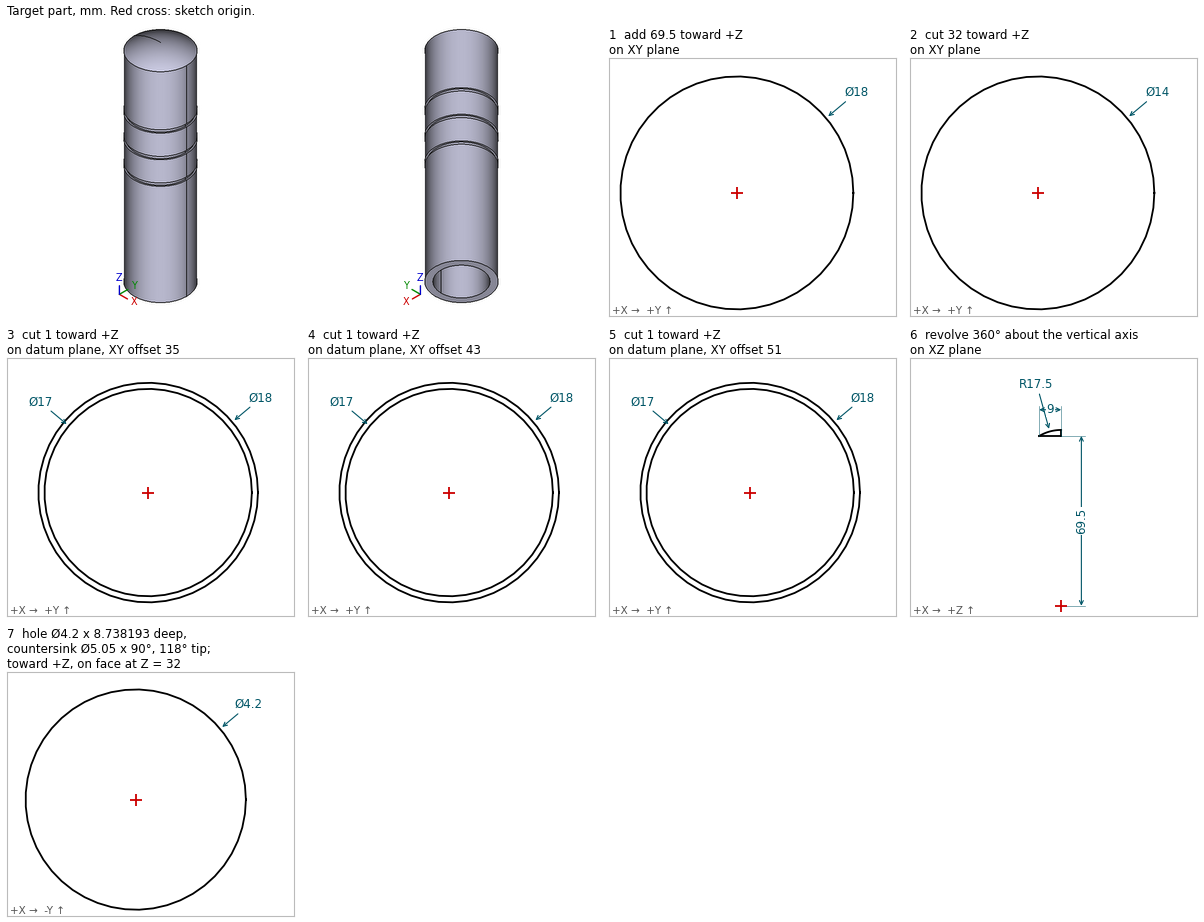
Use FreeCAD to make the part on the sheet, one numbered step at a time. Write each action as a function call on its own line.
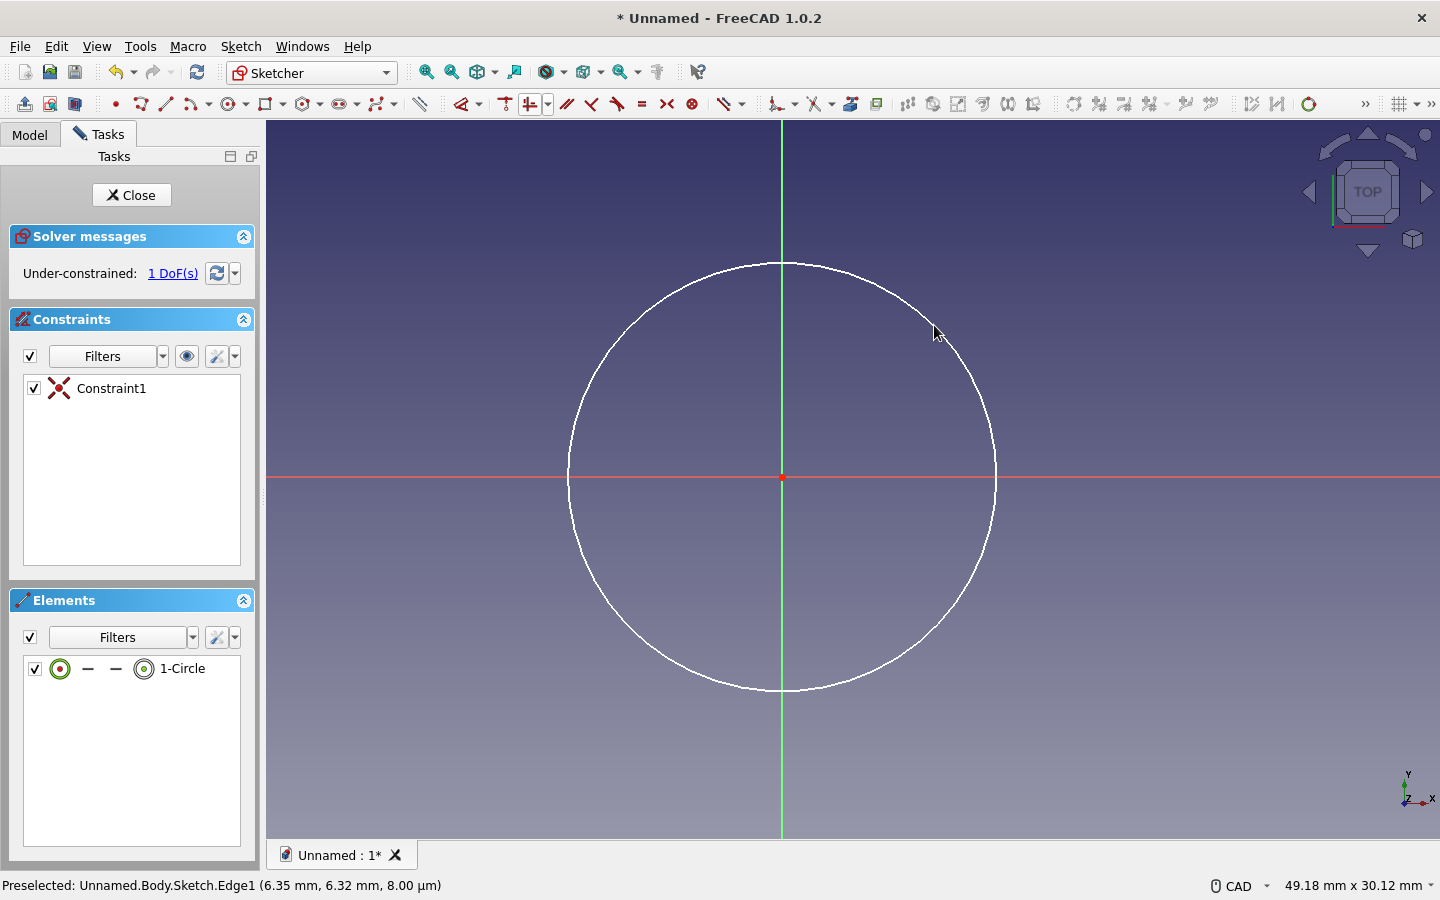
click(460, 104)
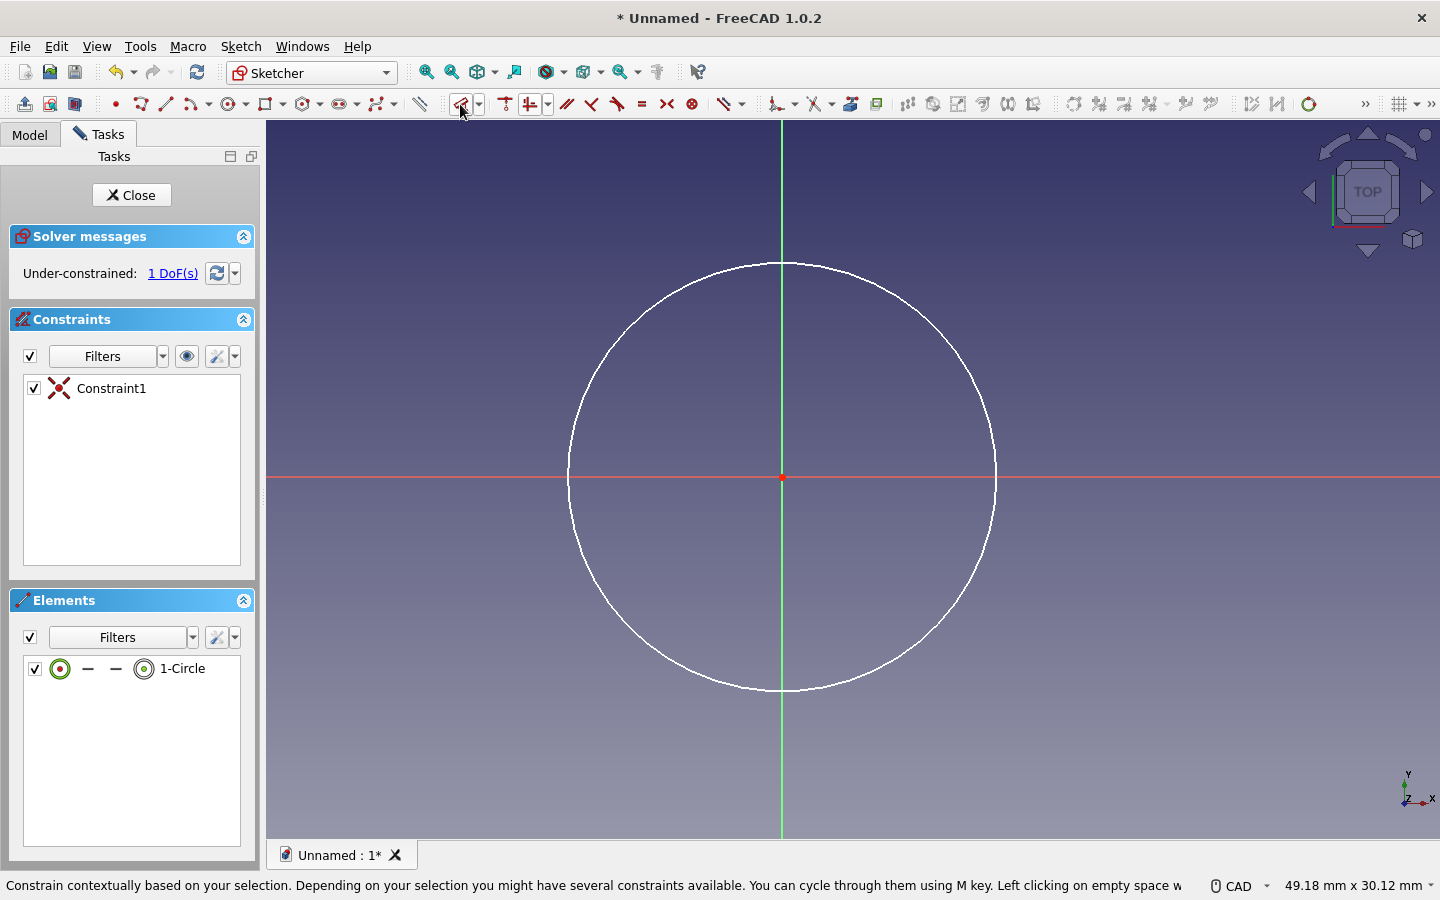
click(933, 325)
click(956, 302)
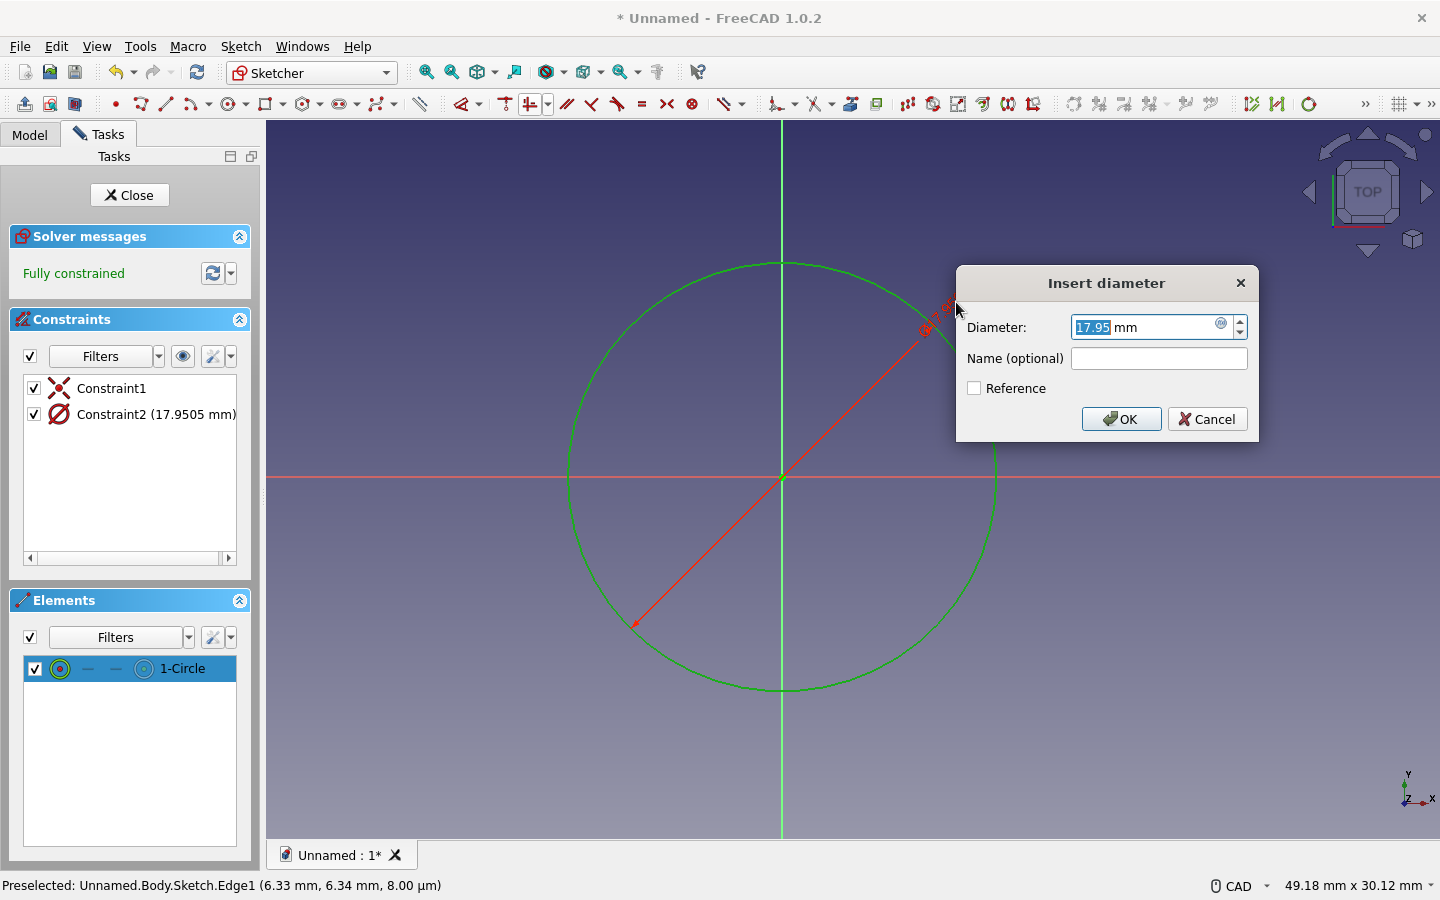
text(18)
key(Return)
key(Escape)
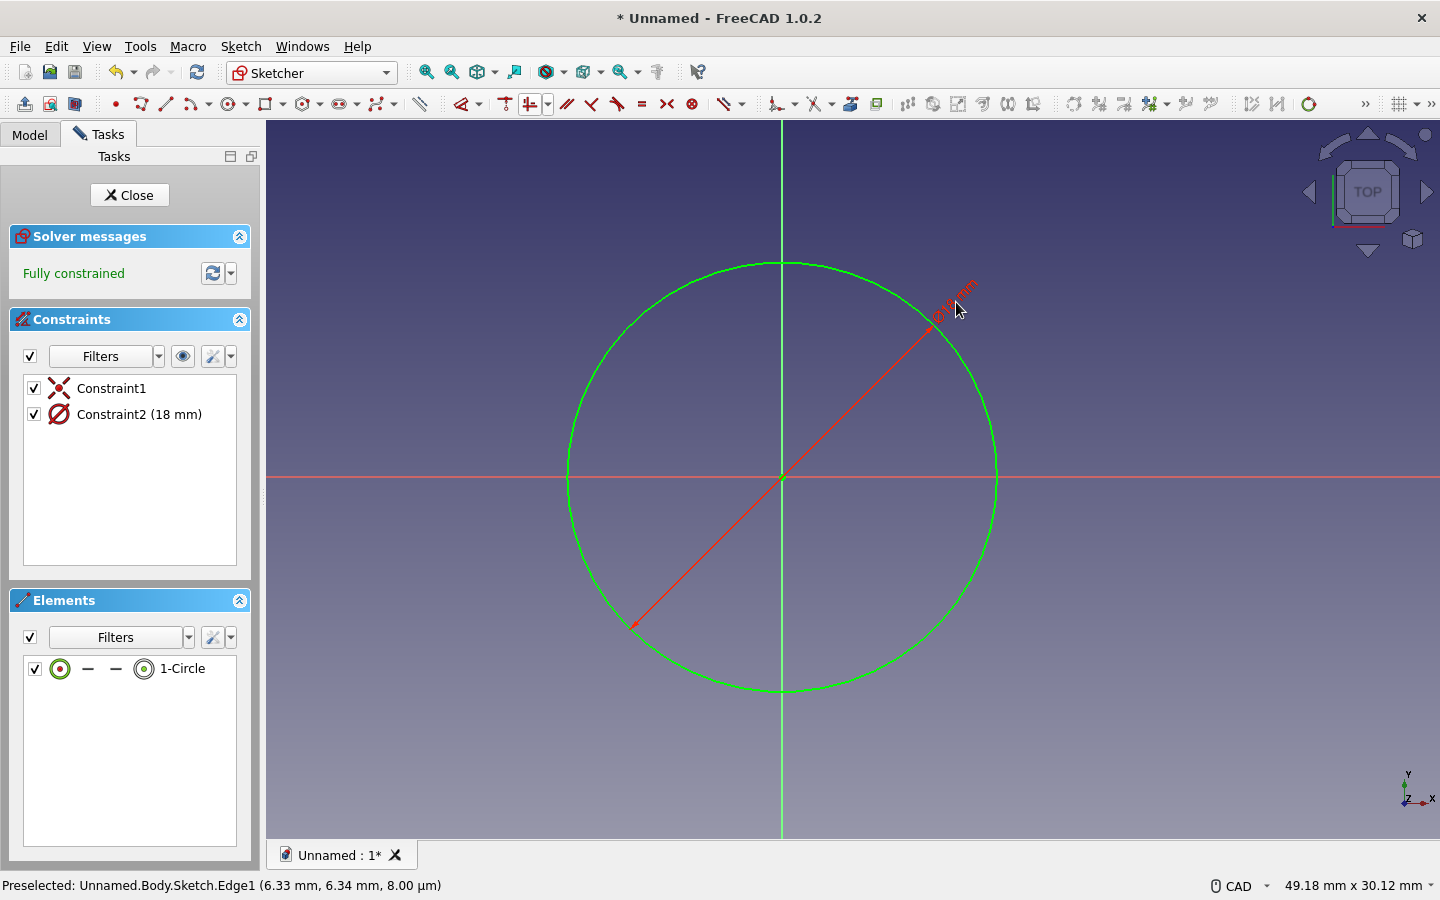
click(130, 195)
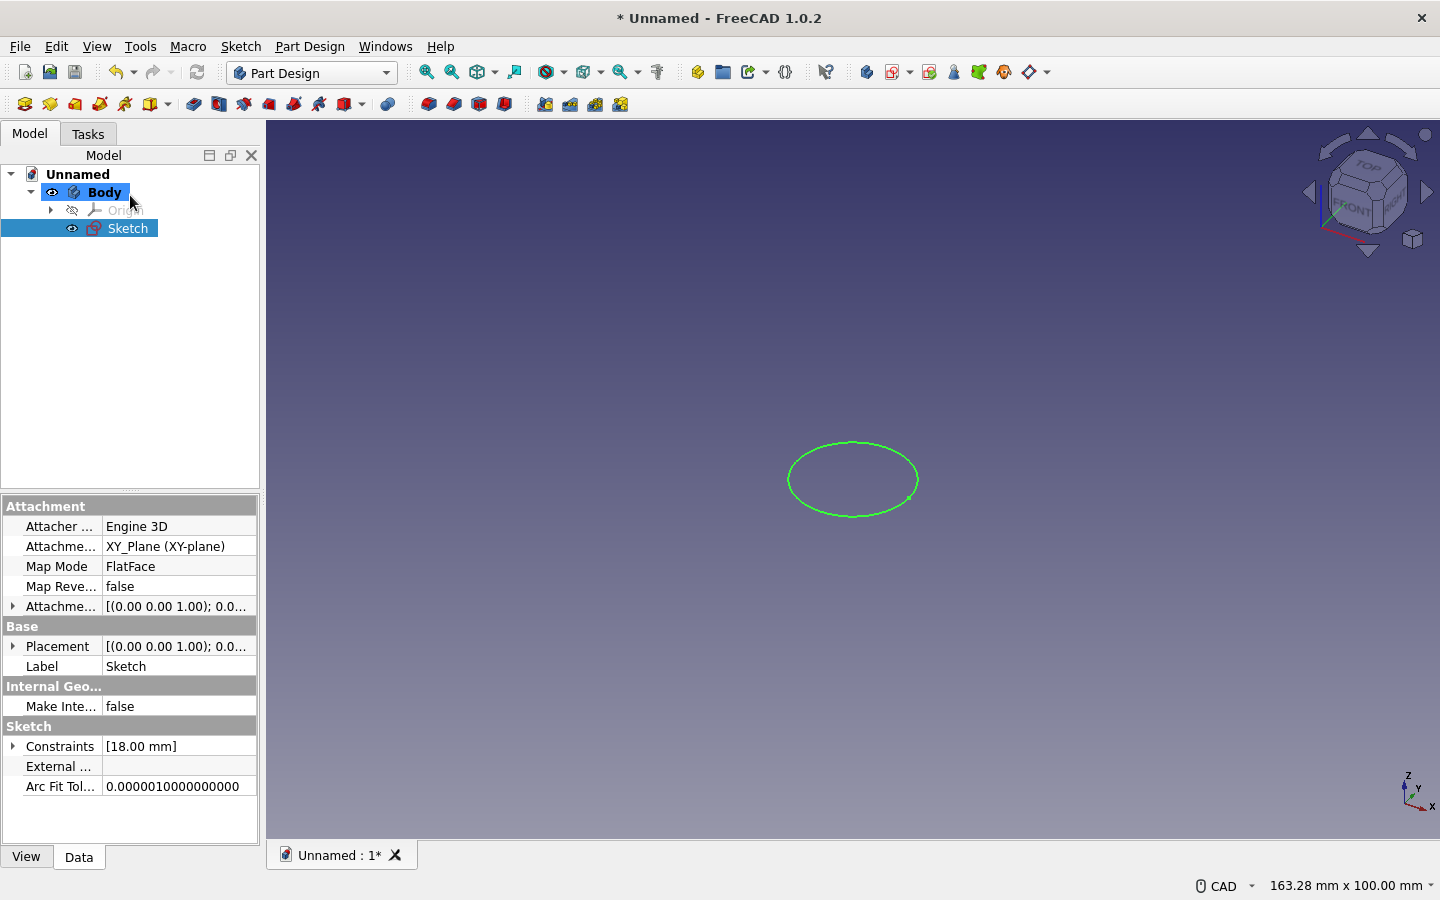
click(25, 104)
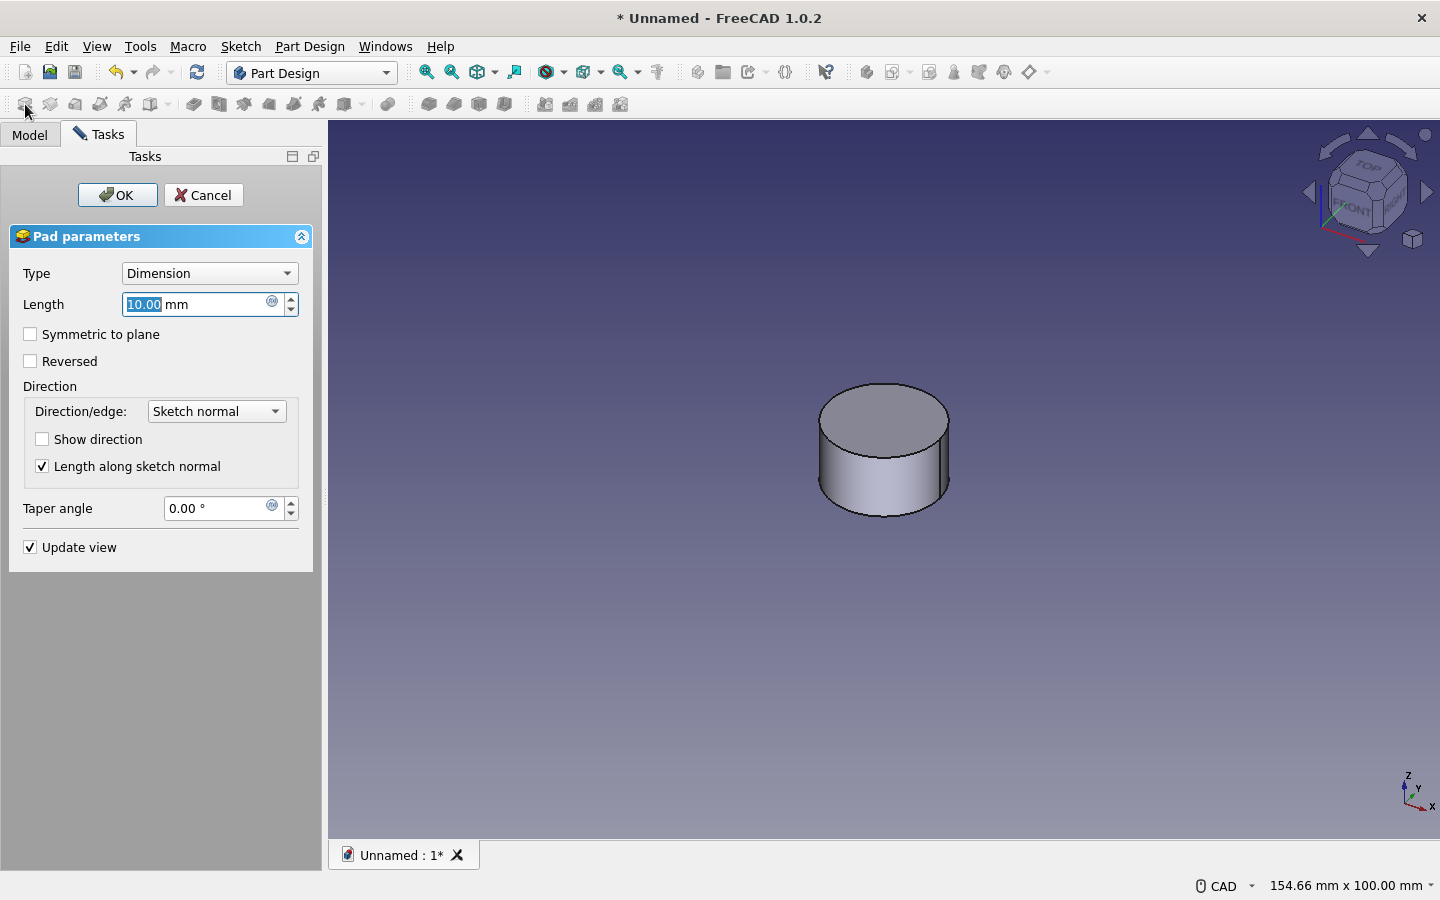
text(69.5)
key(Tab)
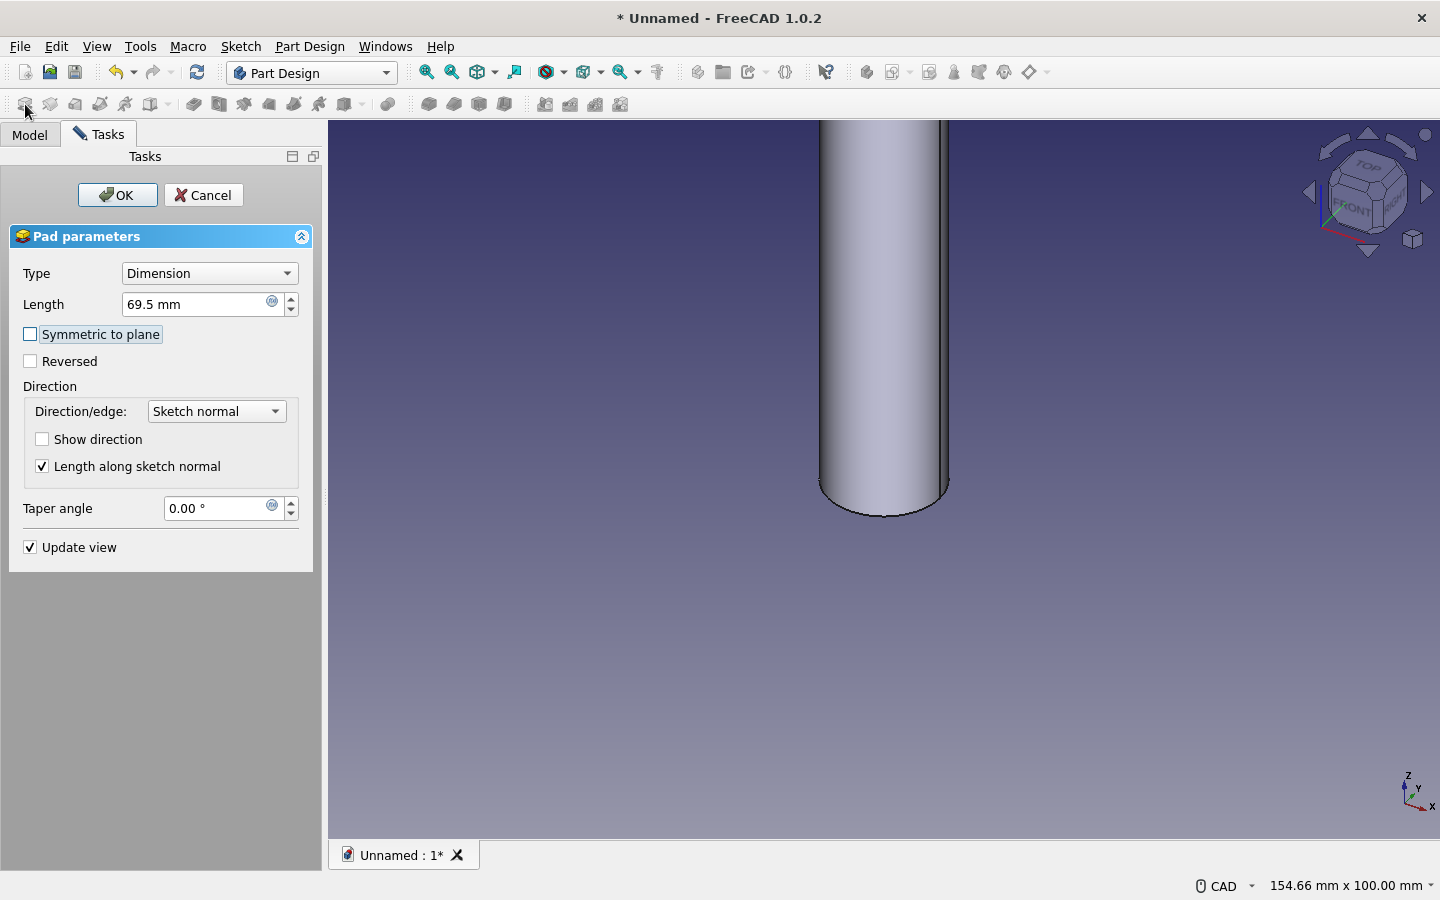
click(118, 195)